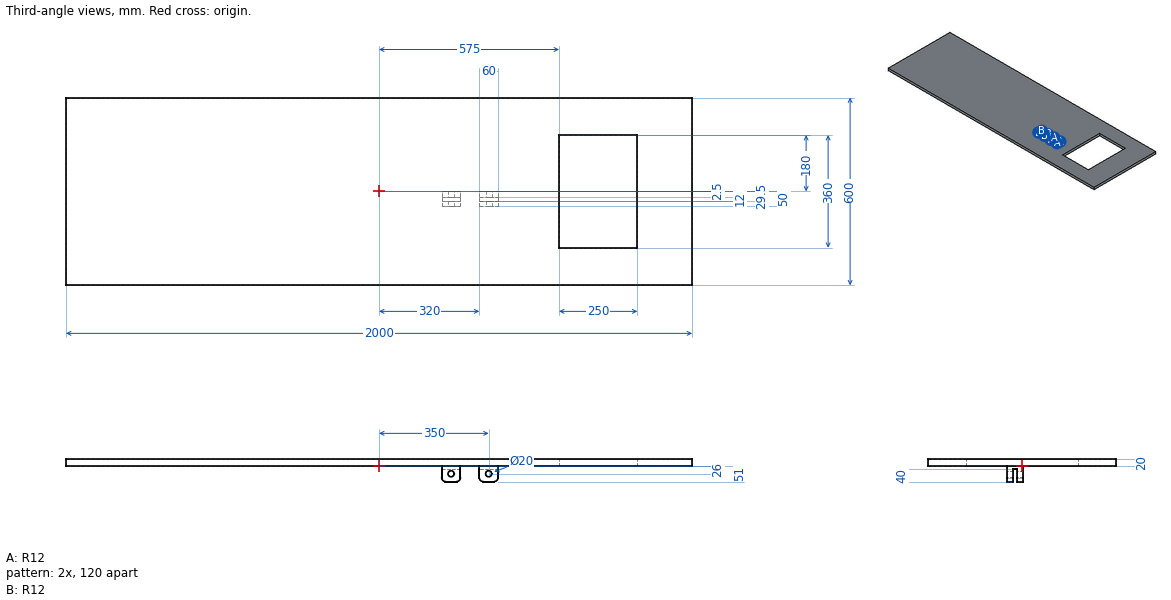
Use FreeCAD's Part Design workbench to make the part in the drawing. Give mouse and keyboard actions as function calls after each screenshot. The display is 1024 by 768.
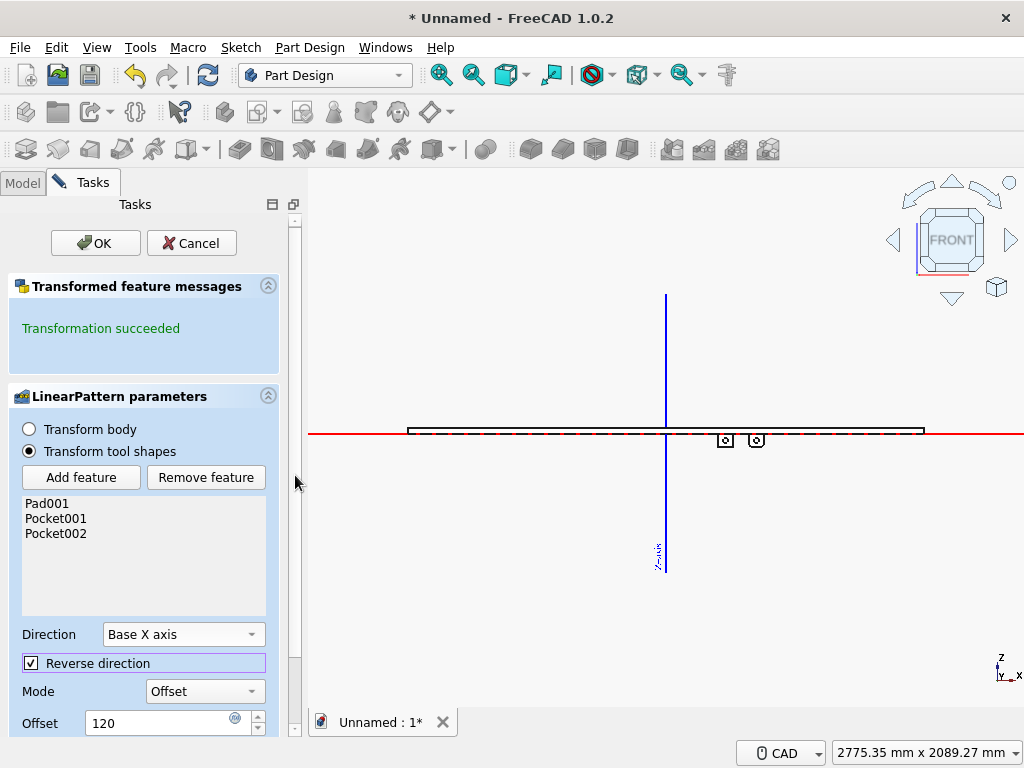
click(96, 243)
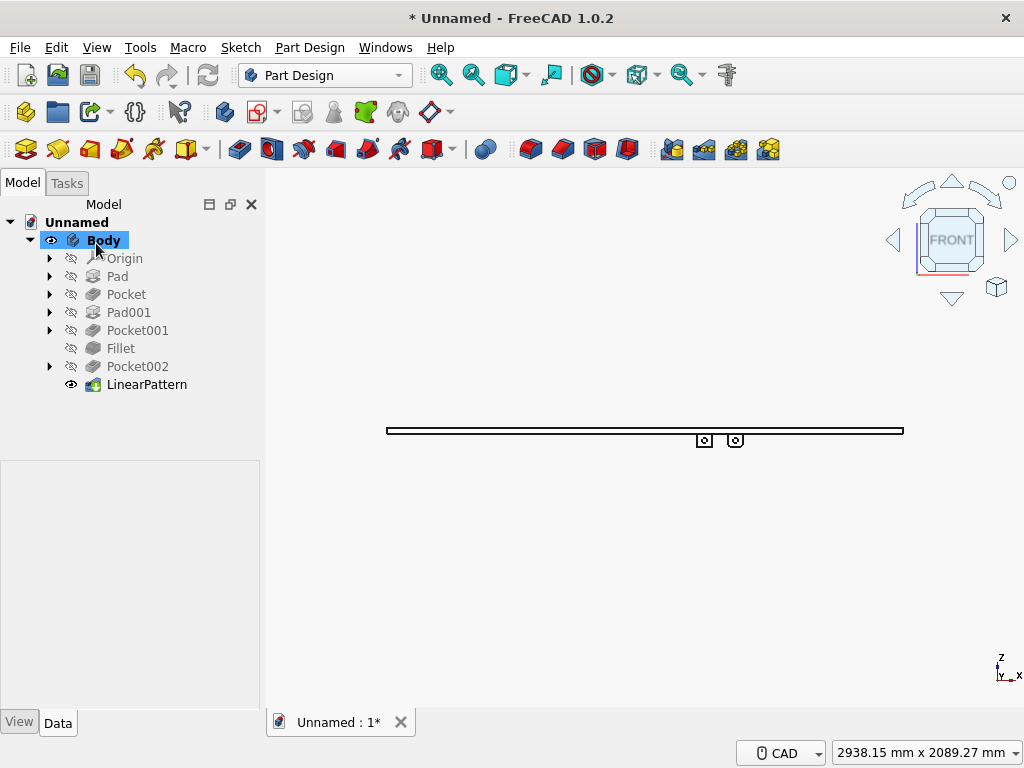
scroll(712, 446, up, 11)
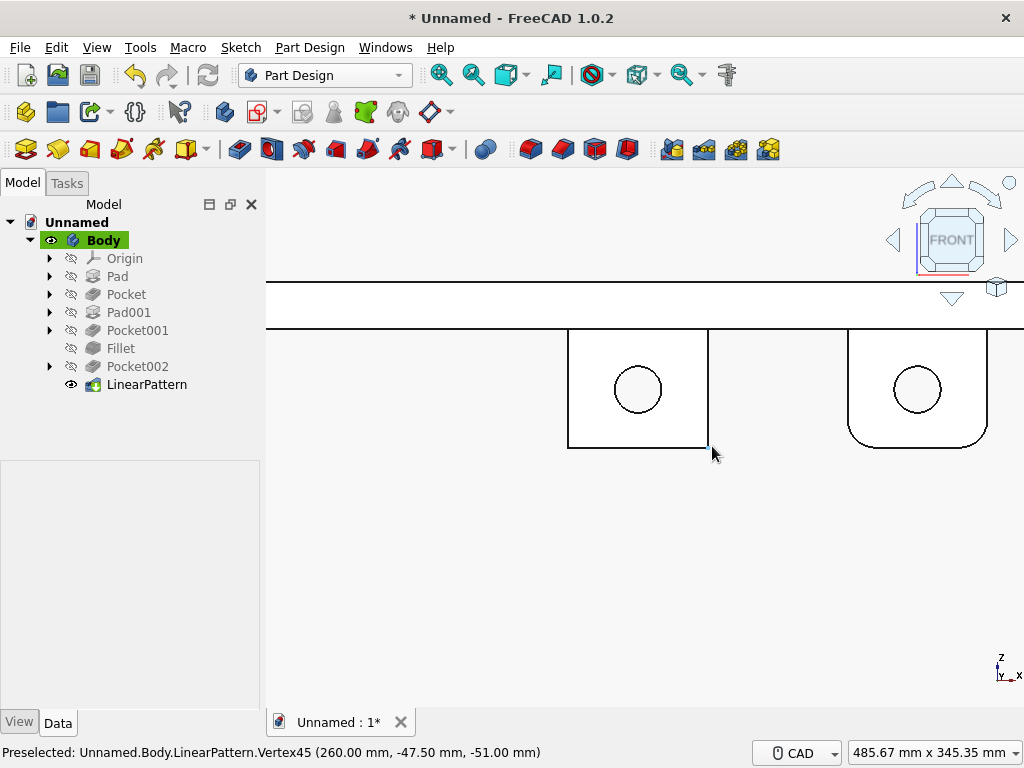
key(v)
key(f)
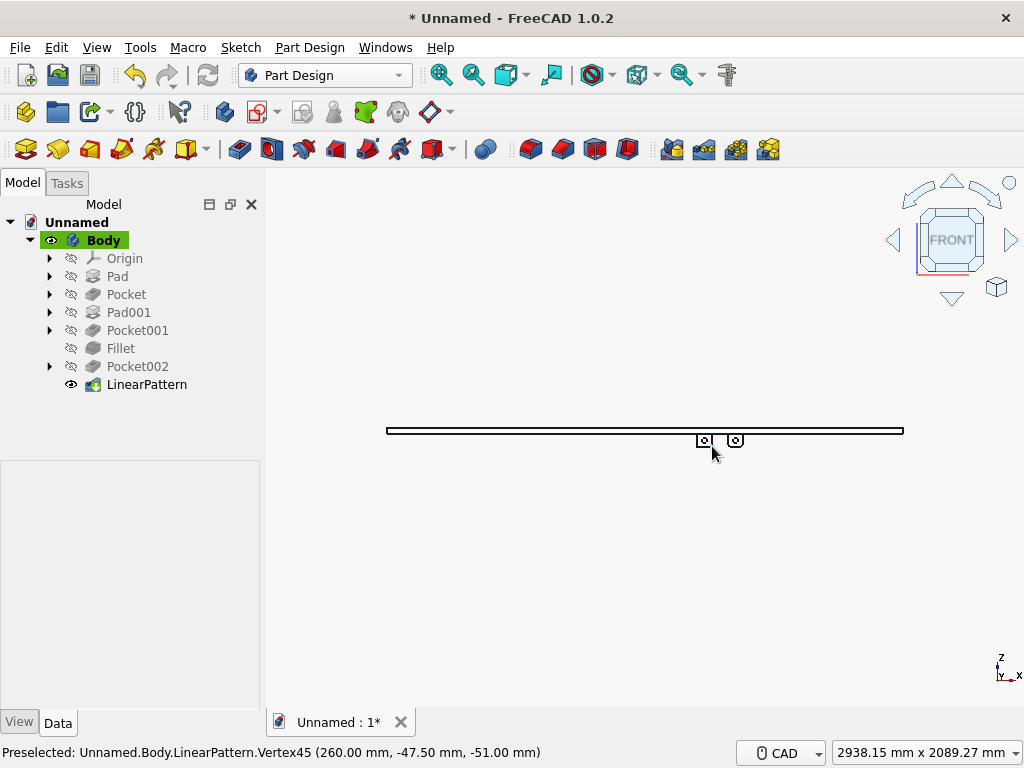
key(0)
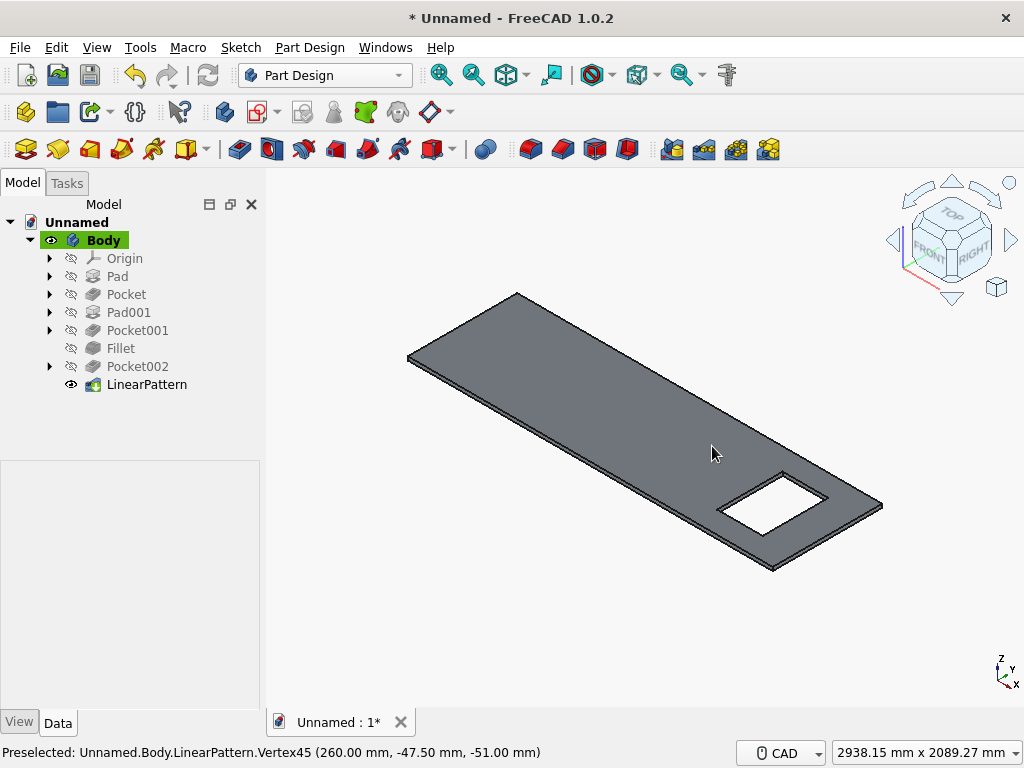
scroll(691, 472, up, 11)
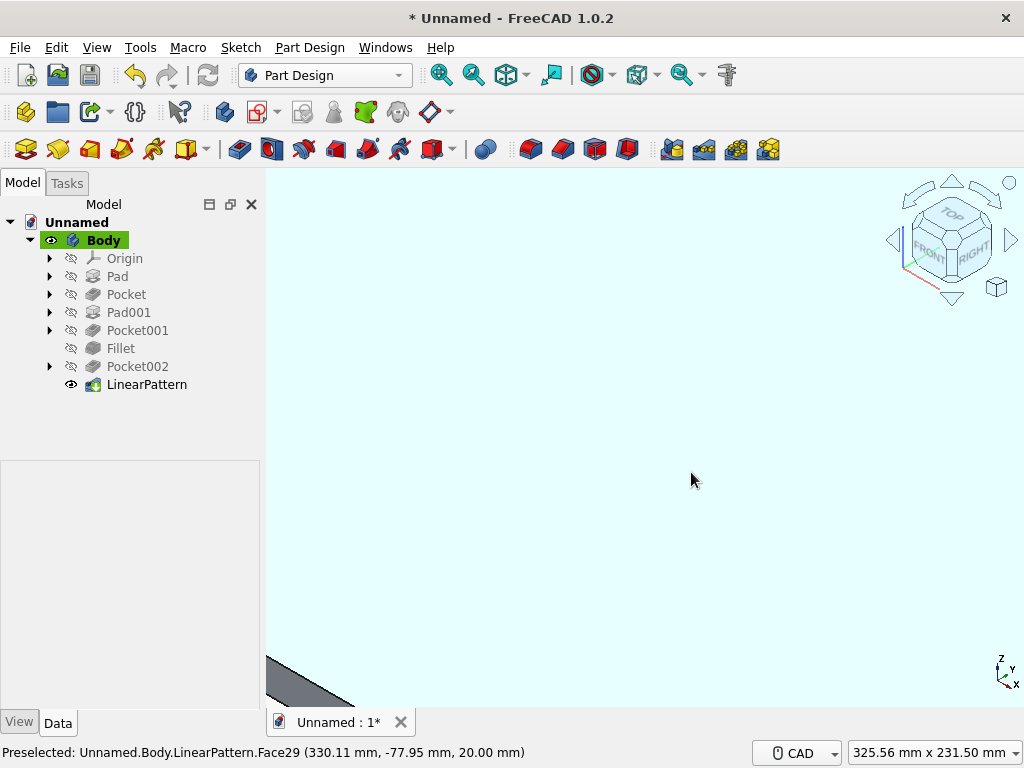
key(v)
key(f)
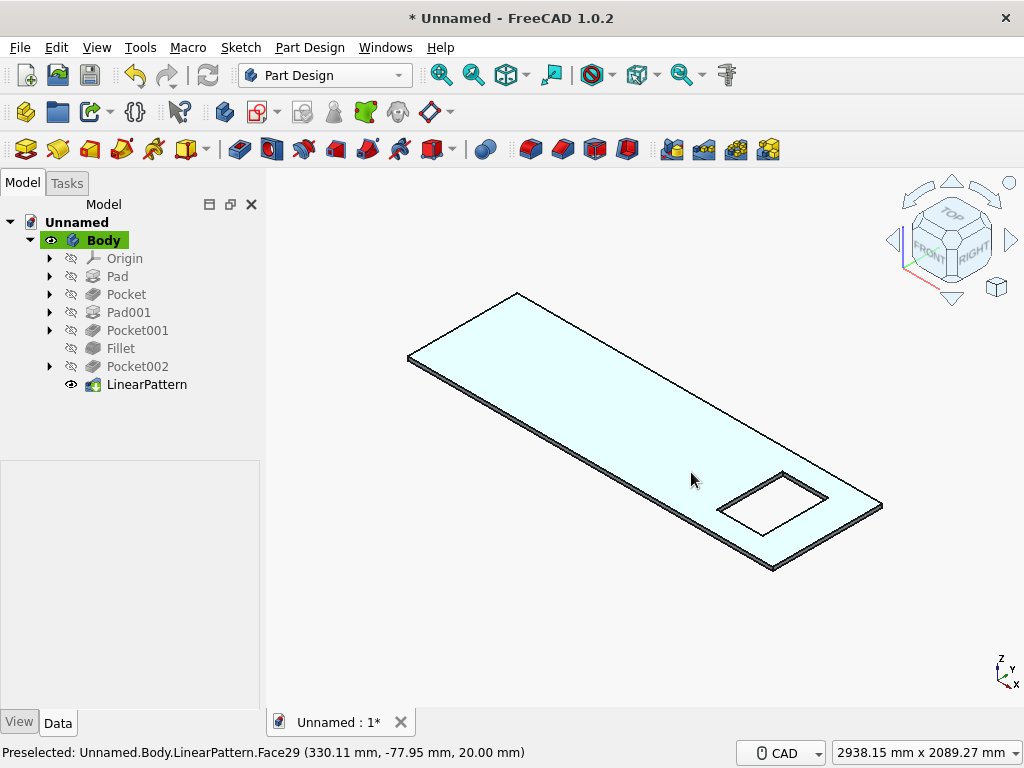
key(2)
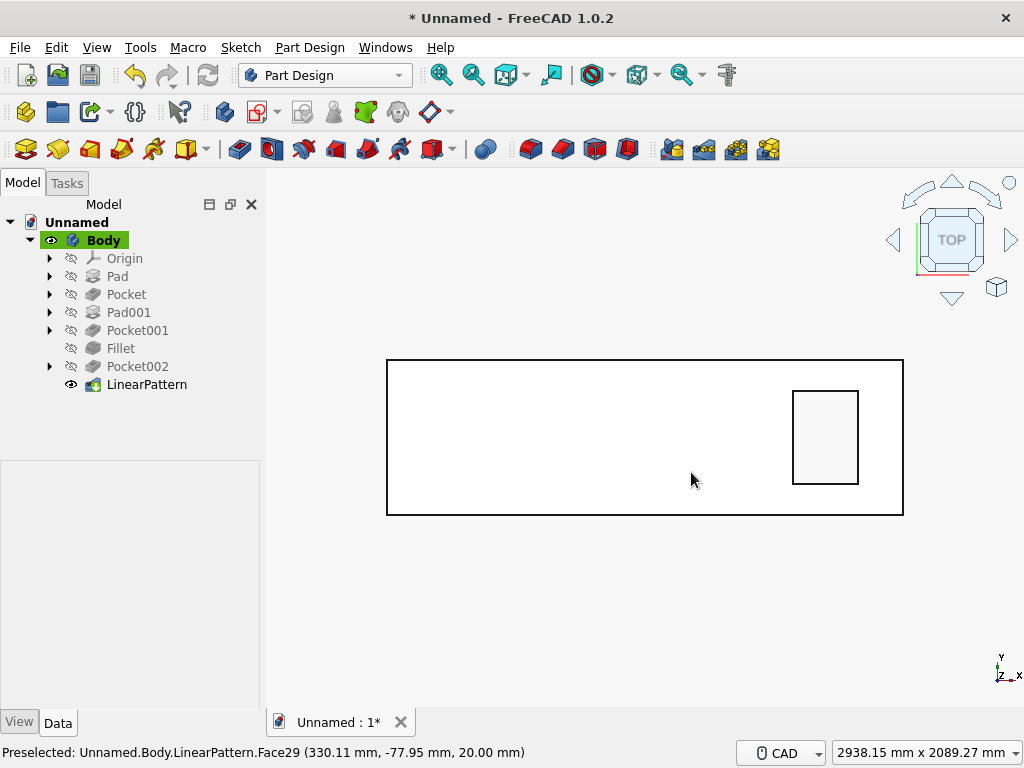
scroll(712, 438, up, 11)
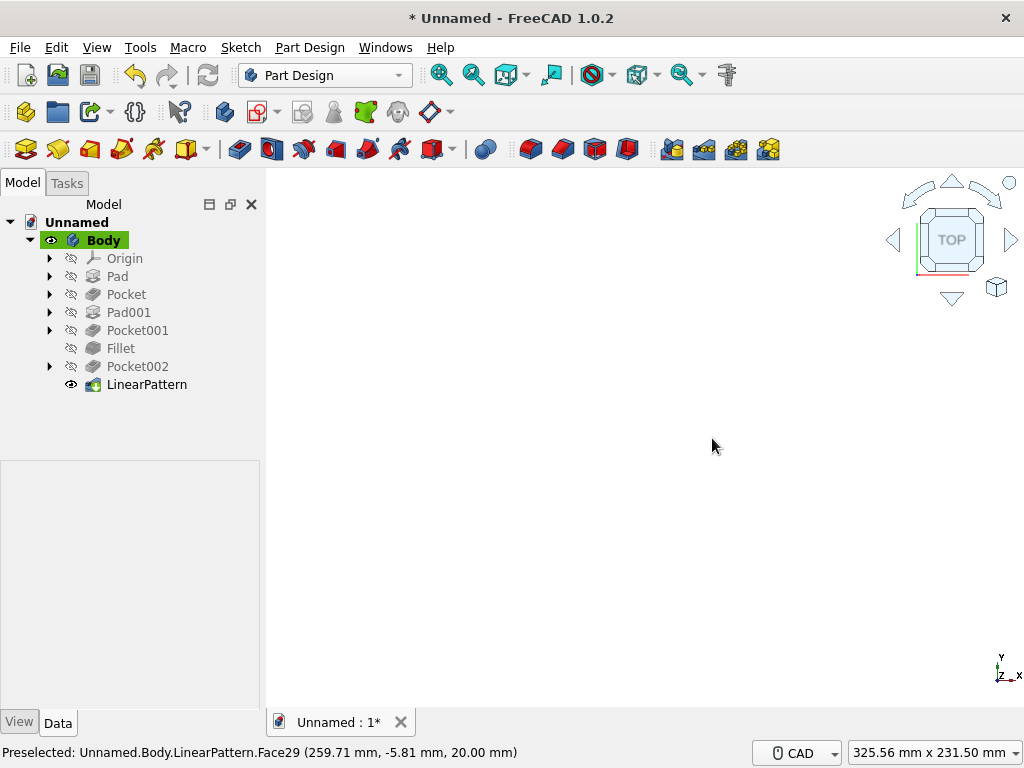
click(442, 76)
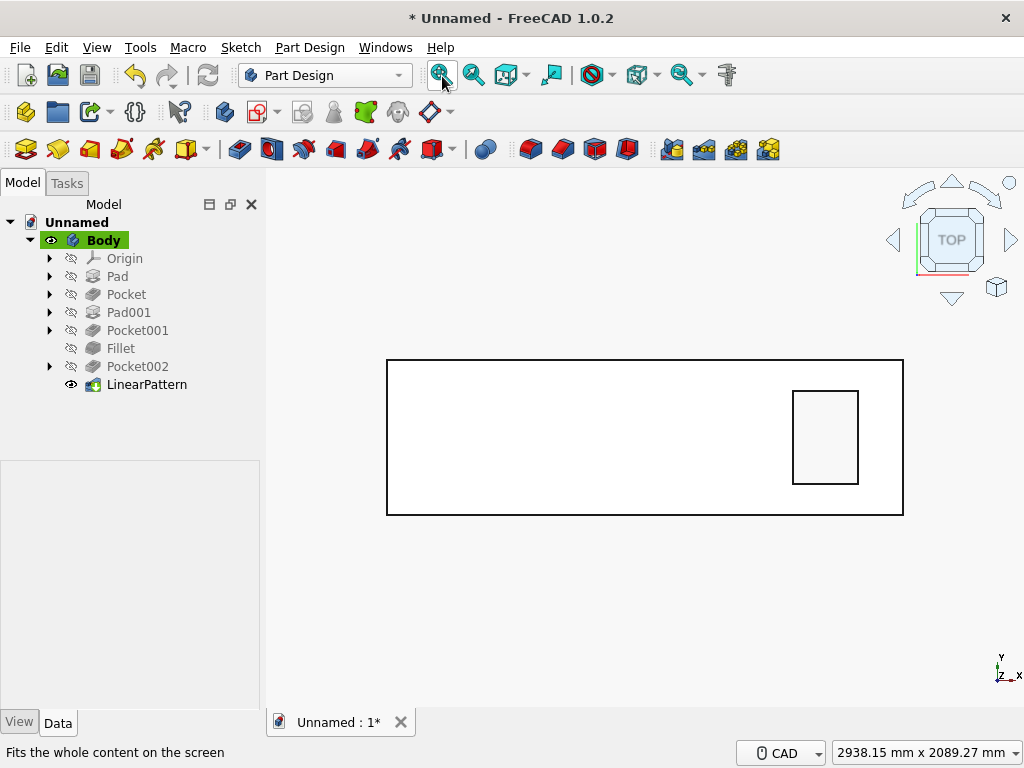
key(1)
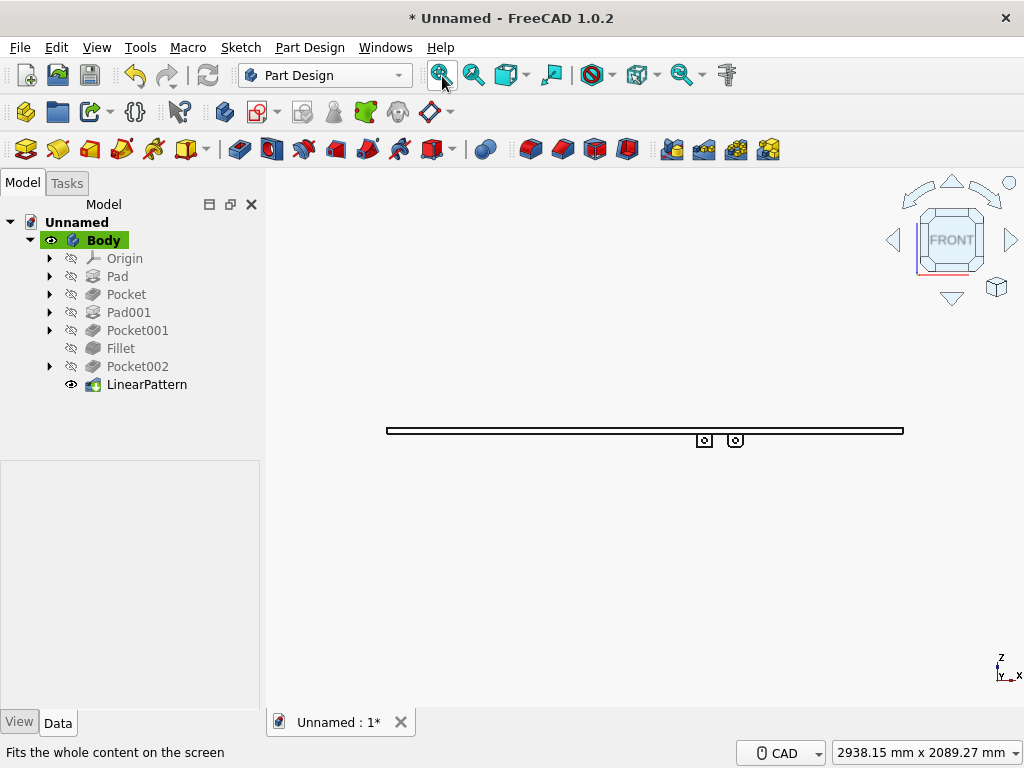
scroll(712, 446, up, 11)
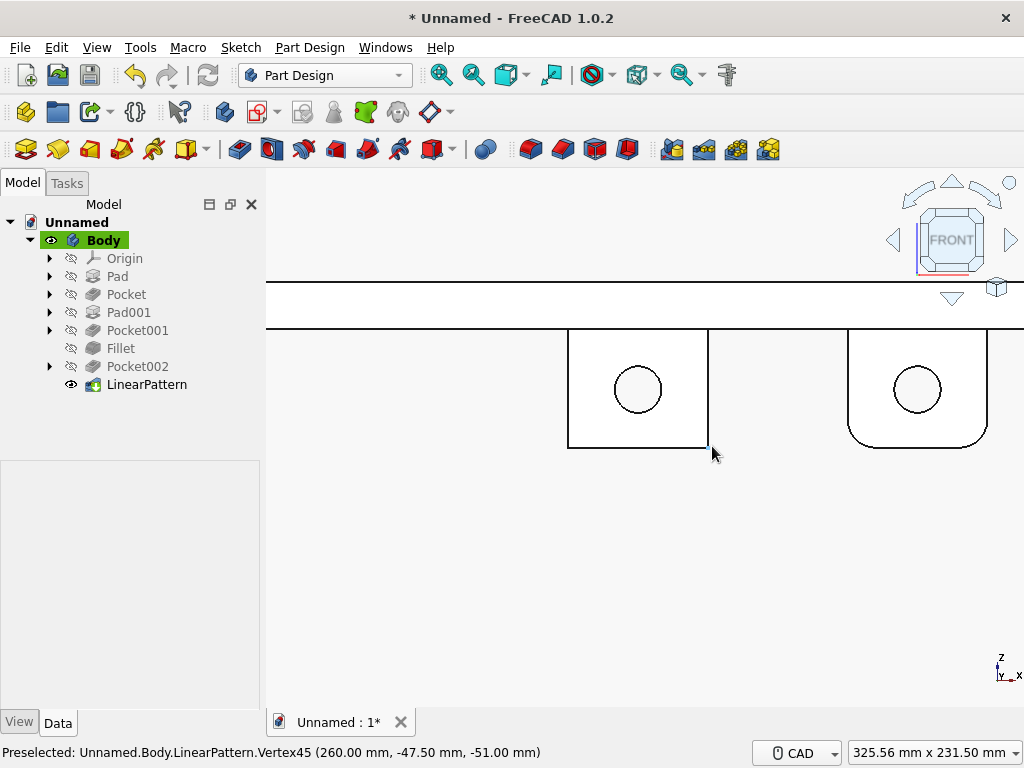
key(v)
key(f)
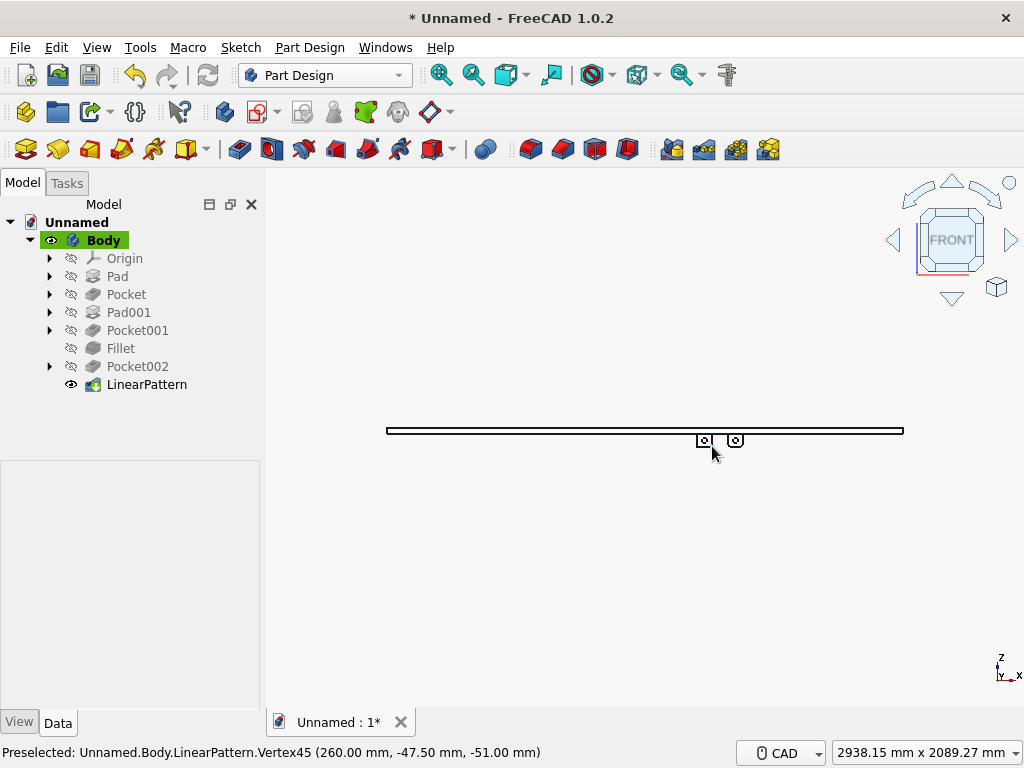
key(3)